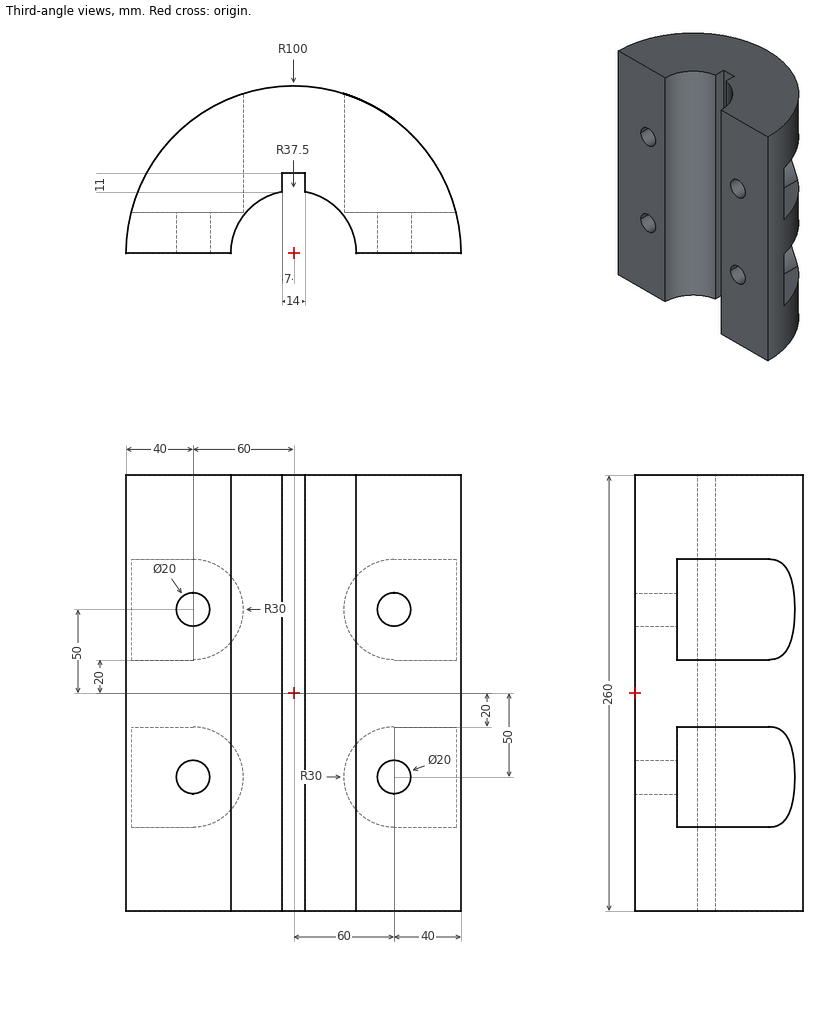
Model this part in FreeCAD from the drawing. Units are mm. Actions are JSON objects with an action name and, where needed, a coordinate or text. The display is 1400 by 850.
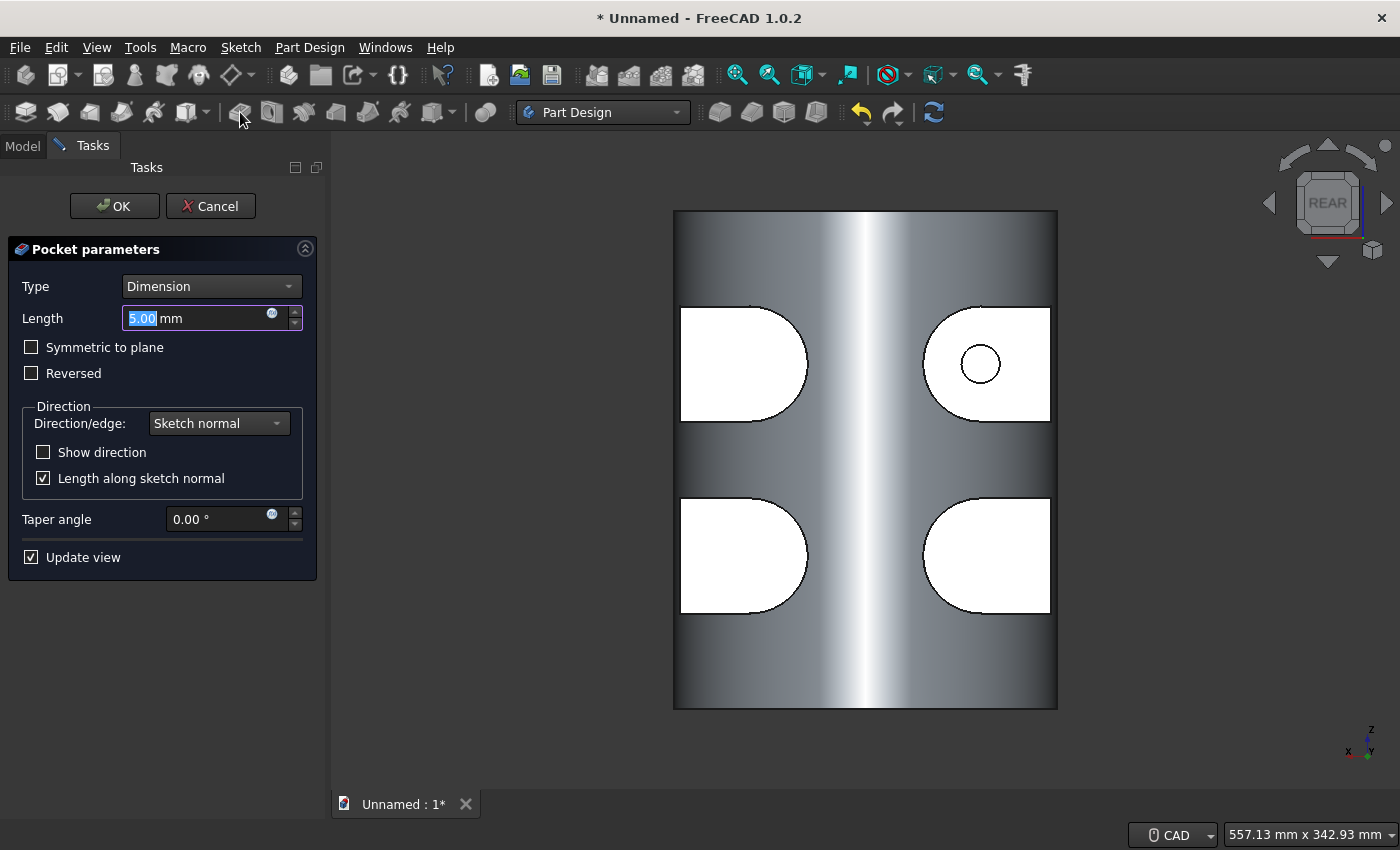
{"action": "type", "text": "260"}
{"action": "key", "text": "Tab"}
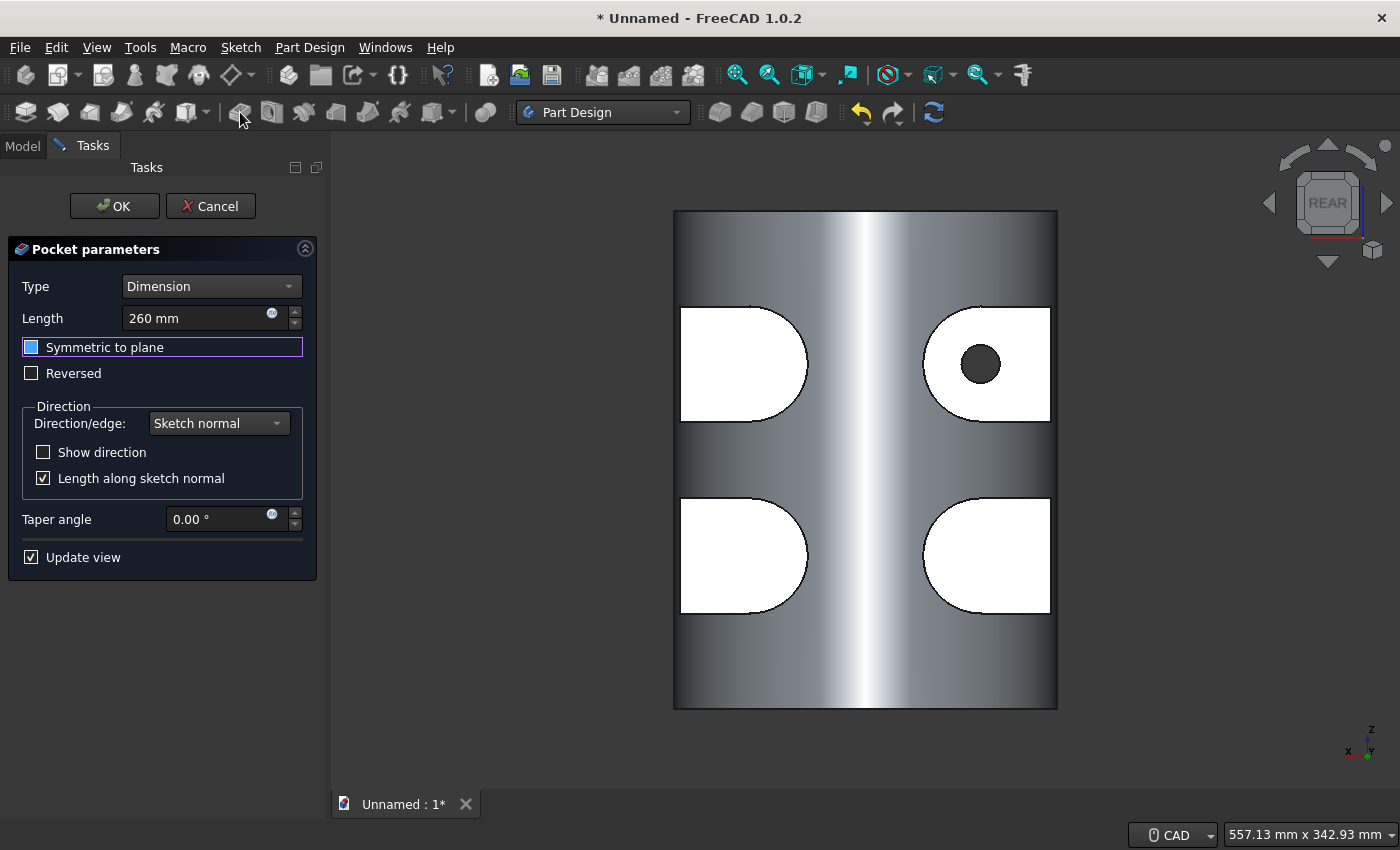
{"action": "left_click", "coordinate": [115, 206]}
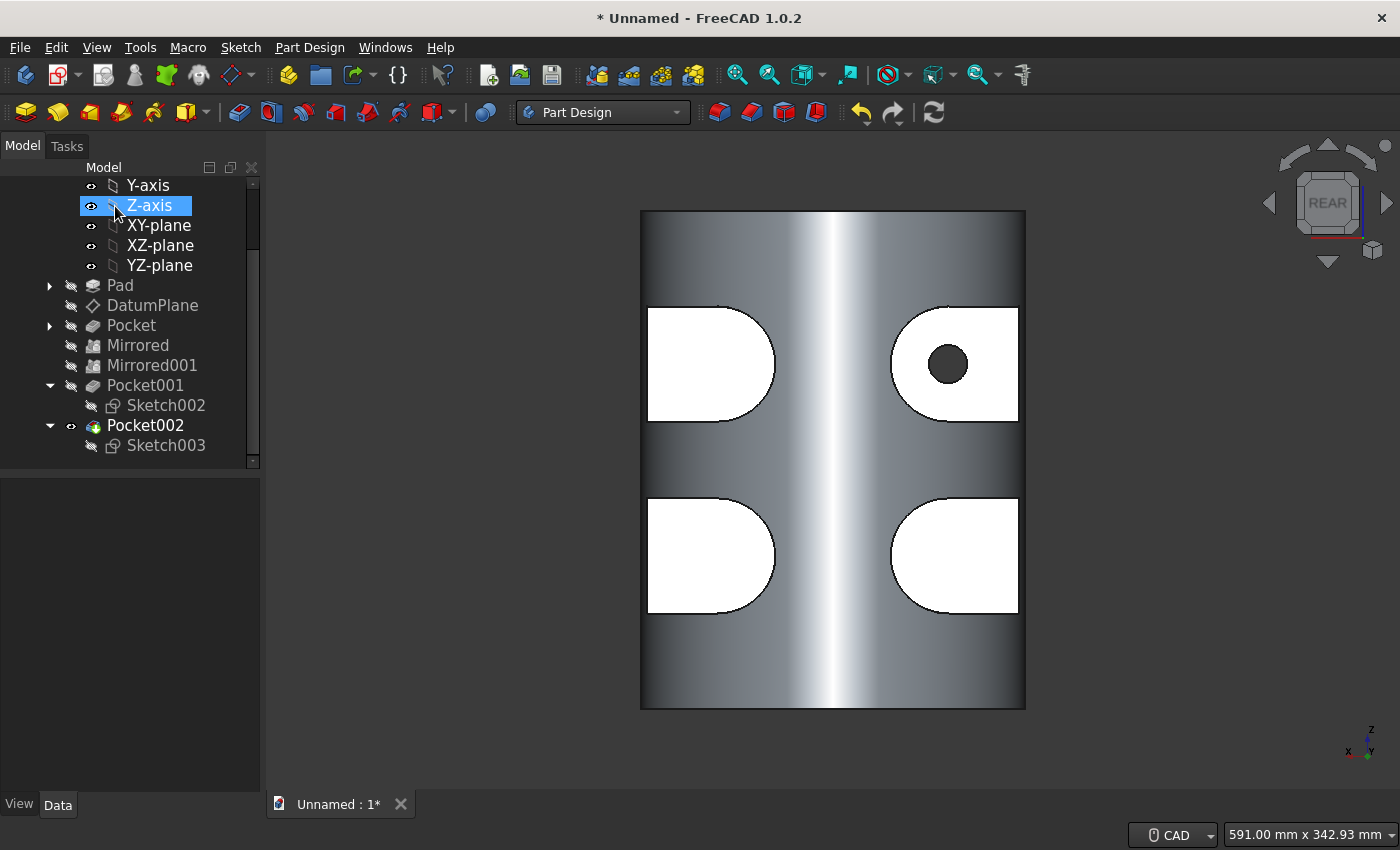
{"action": "left_click", "coordinate": [116, 426]}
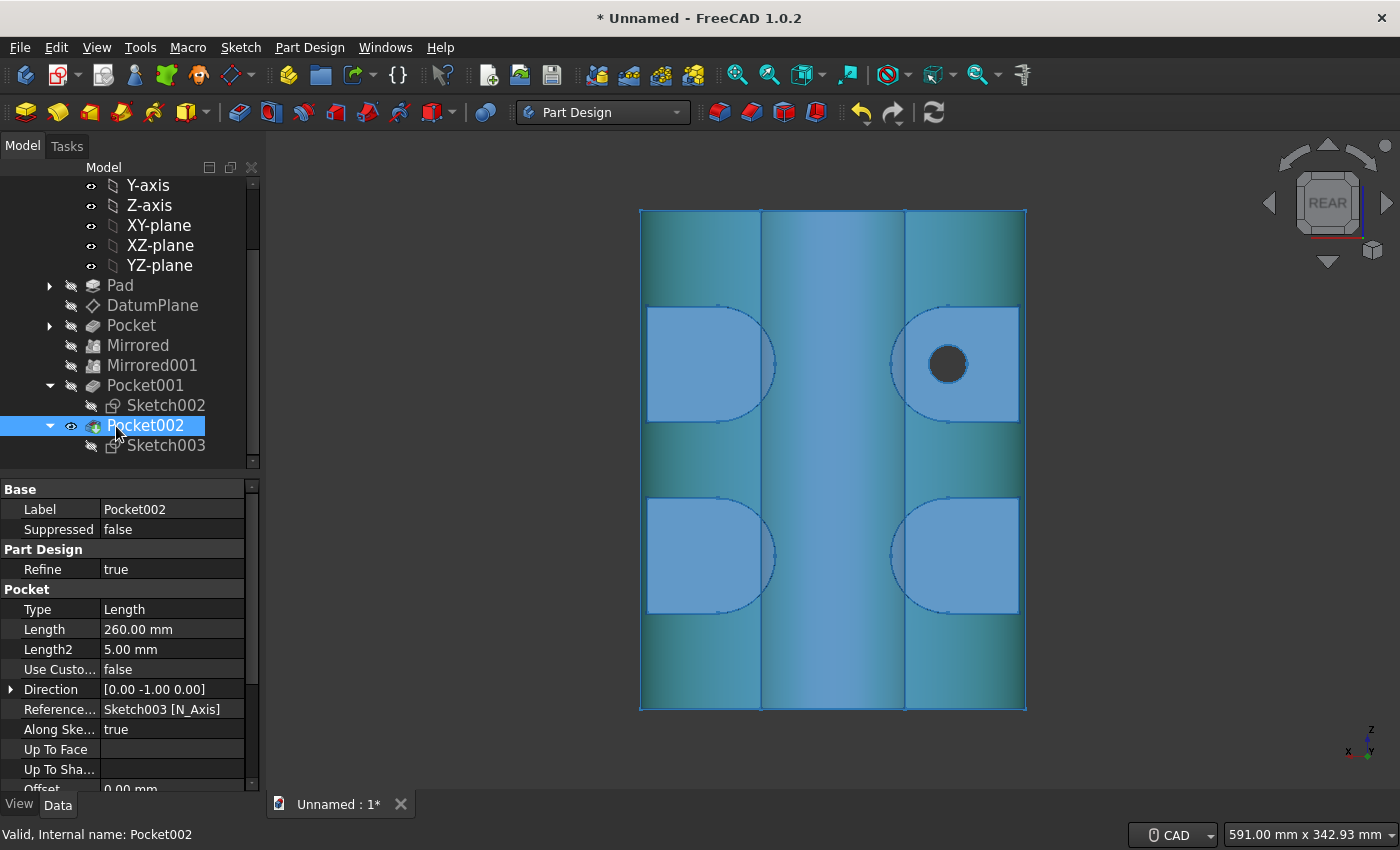
{"action": "left_click", "coordinate": [598, 76]}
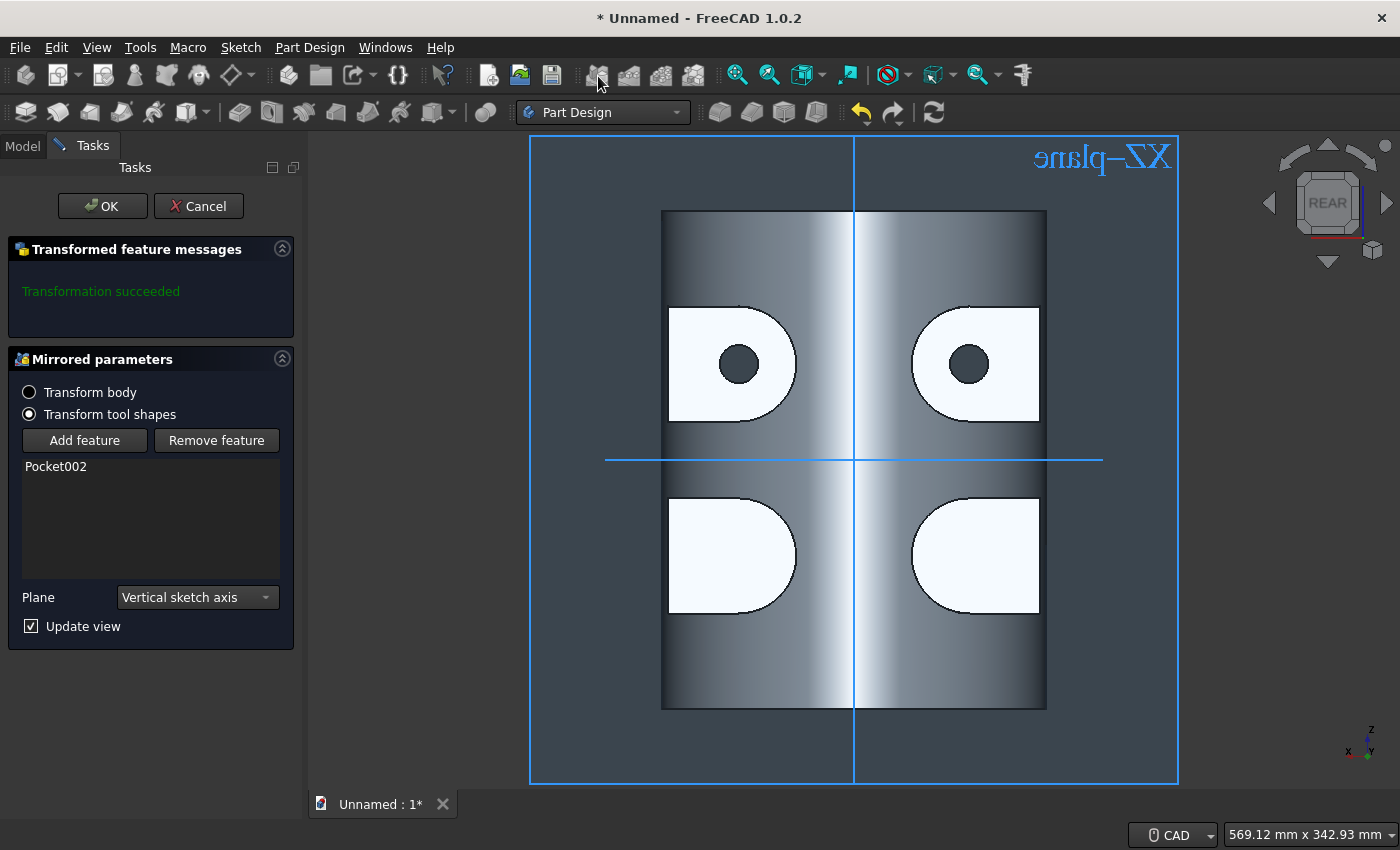
{"action": "left_click", "coordinate": [198, 598]}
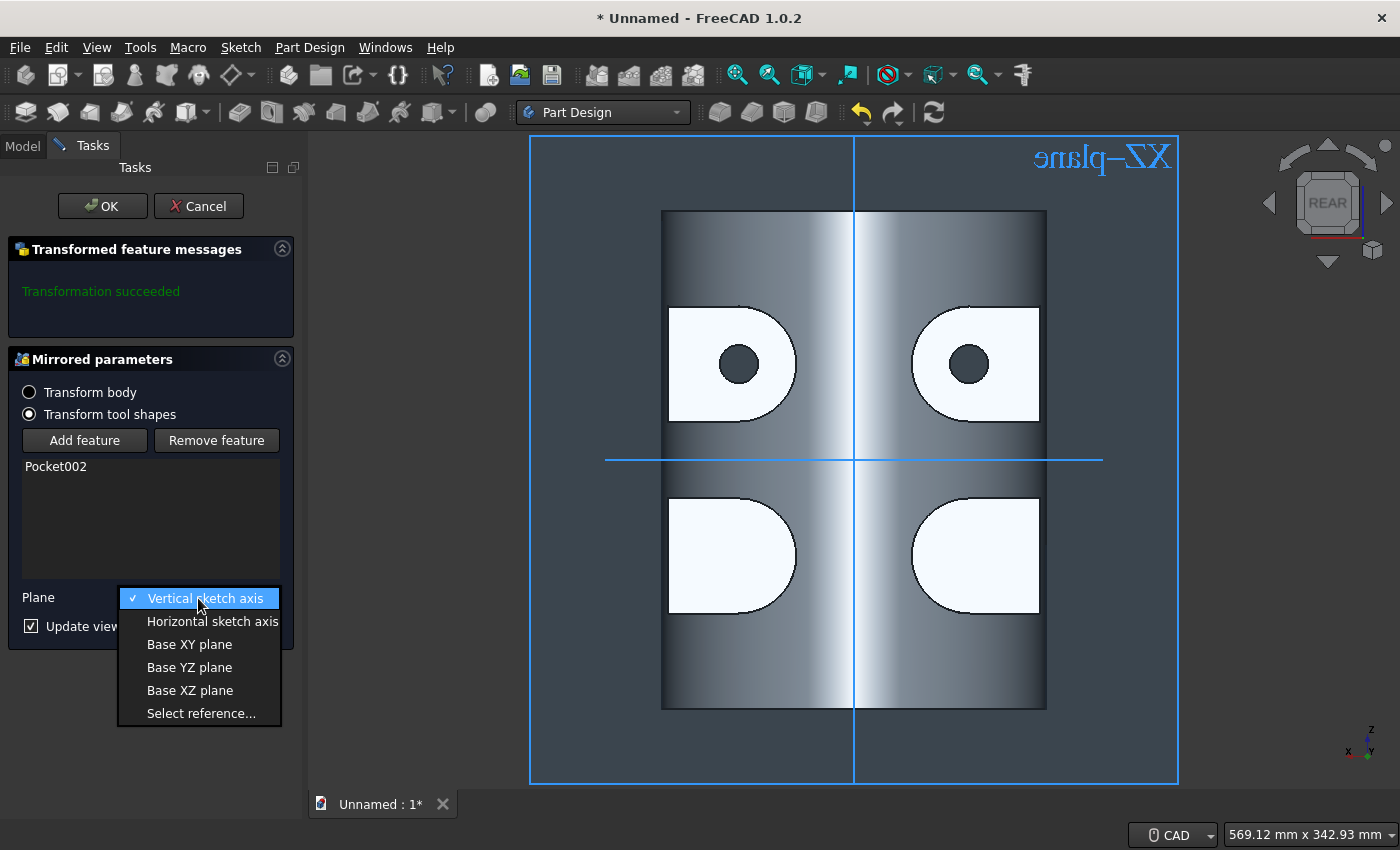
{"action": "left_click", "coordinate": [198, 644]}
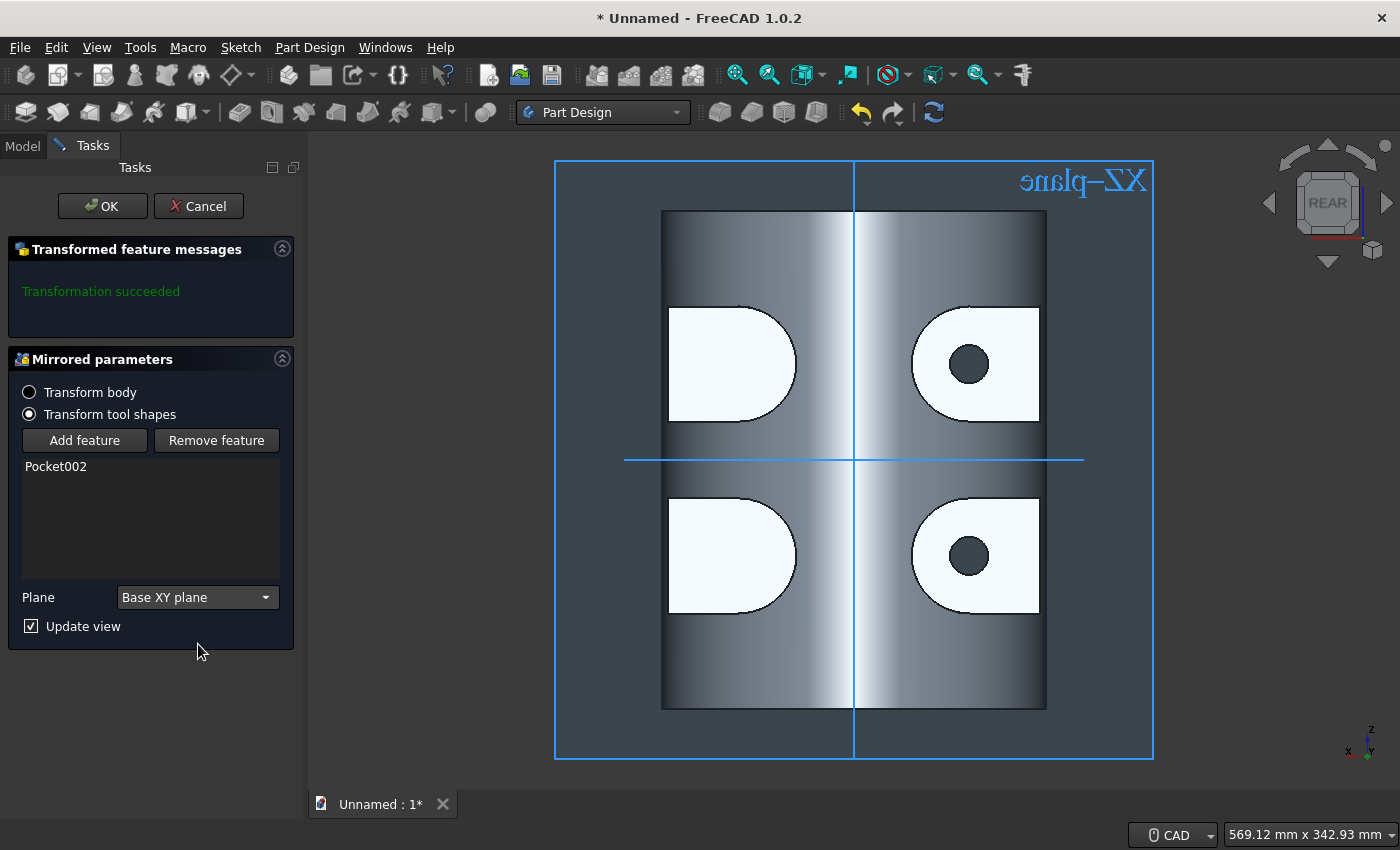
{"action": "left_click", "coordinate": [103, 206]}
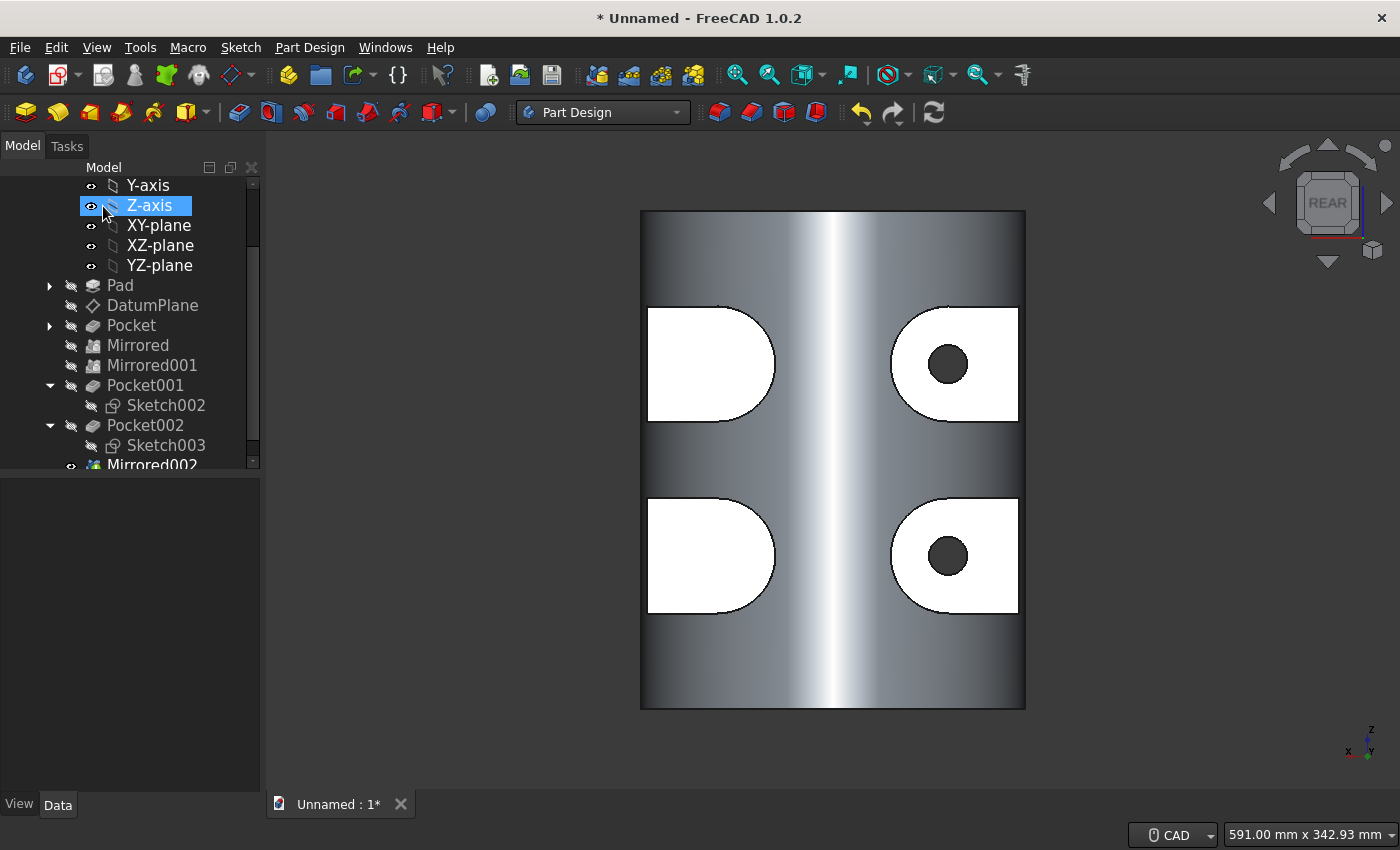
{"action": "left_click", "coordinate": [116, 426]}